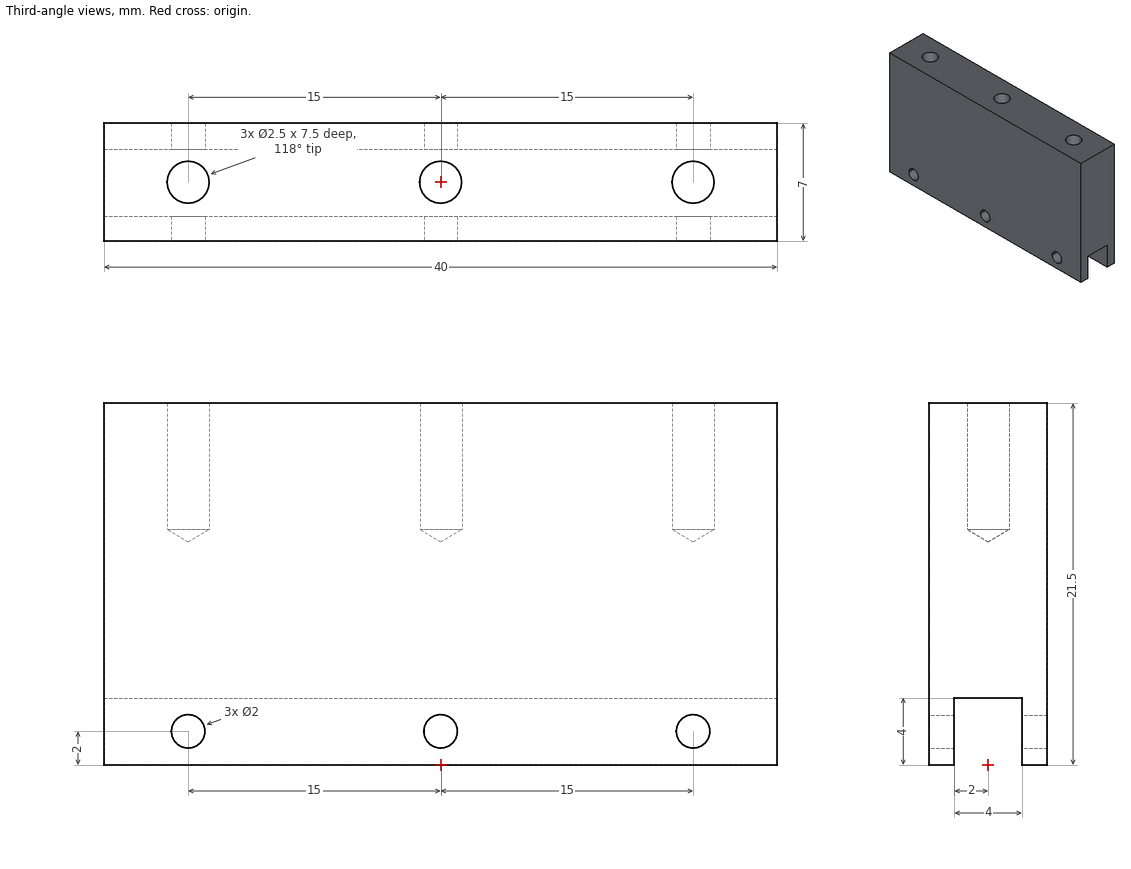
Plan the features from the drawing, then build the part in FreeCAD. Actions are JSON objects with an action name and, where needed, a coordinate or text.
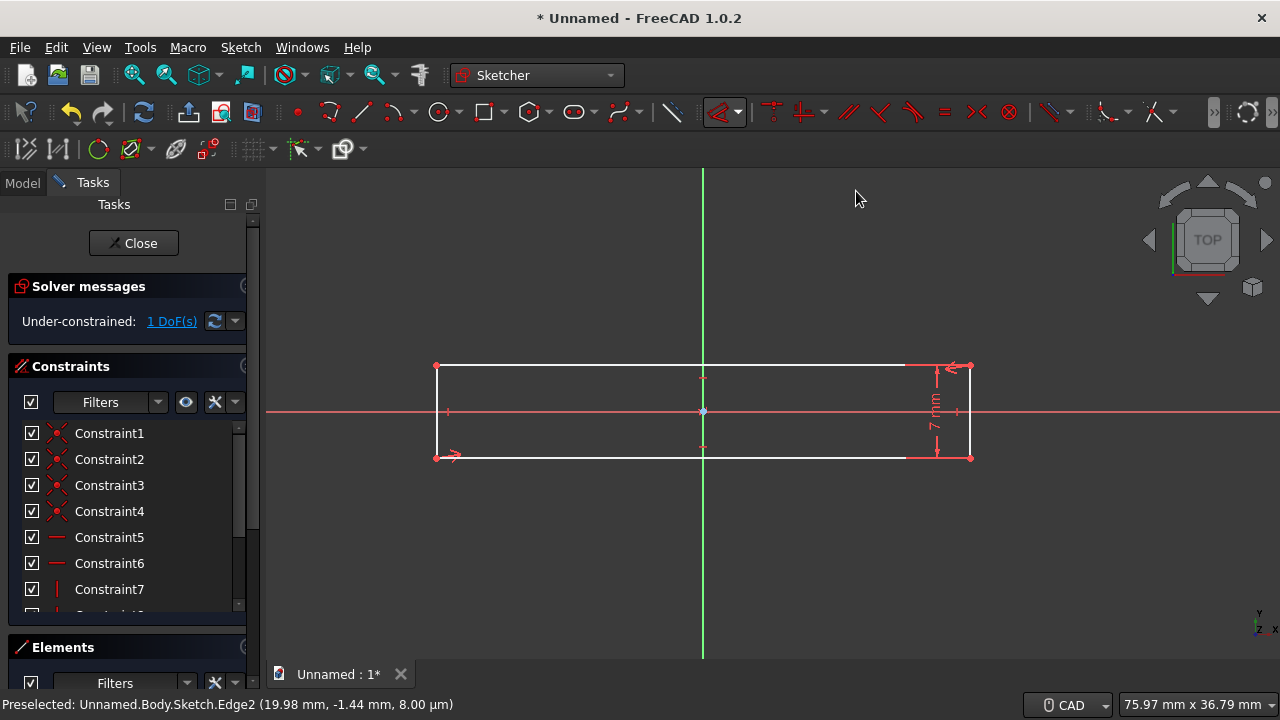
{"action": "left_click", "coordinate": [597, 458]}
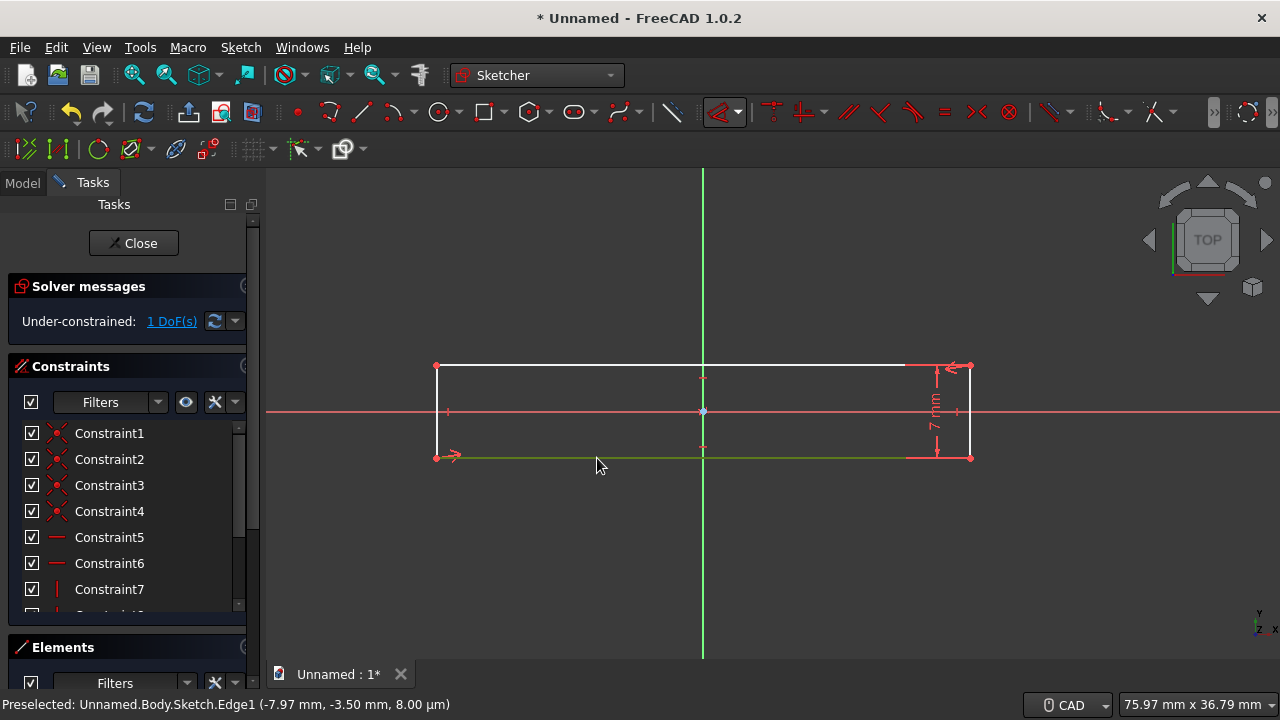
{"action": "left_click", "coordinate": [740, 112]}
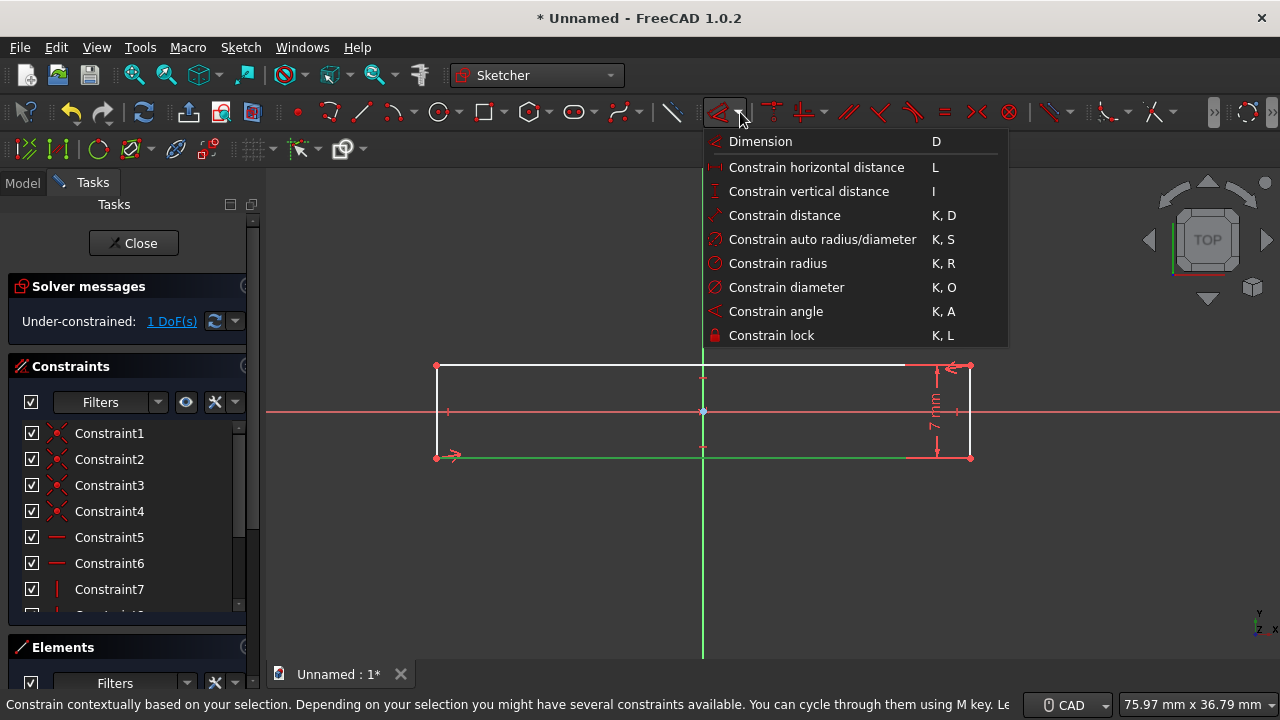
{"action": "left_click", "coordinate": [856, 167]}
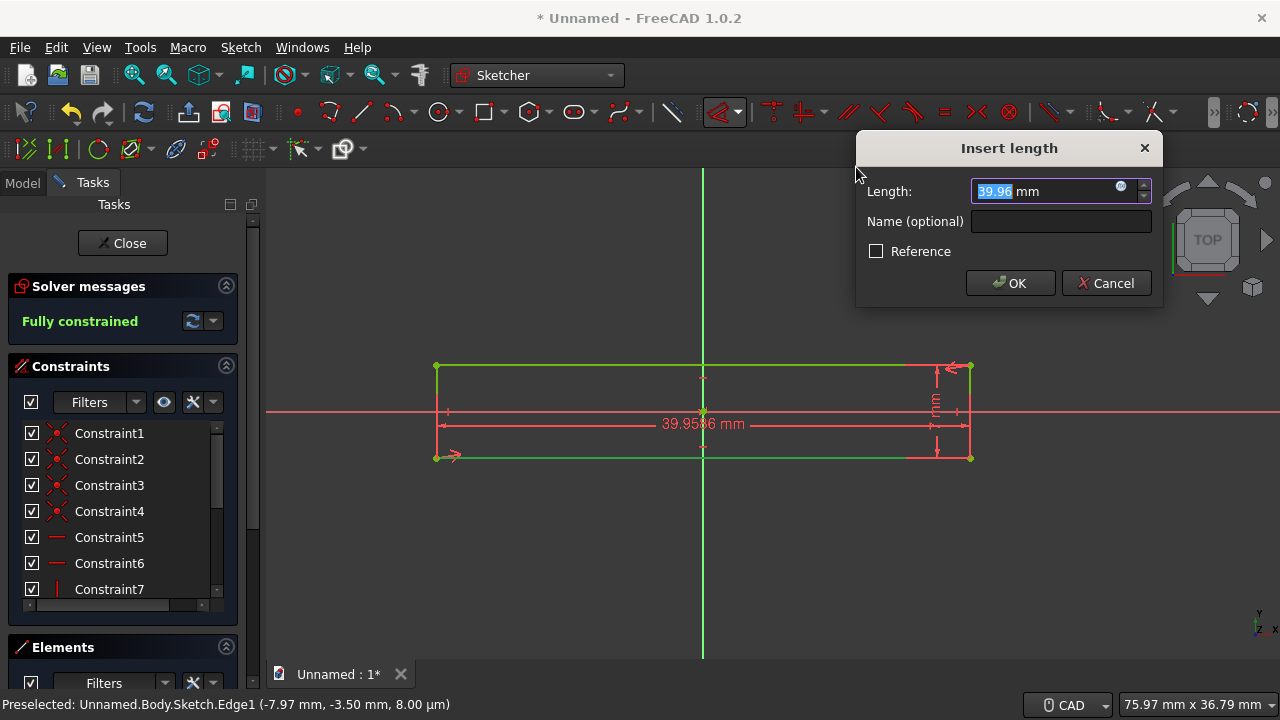
{"action": "type", "text": "40"}
{"action": "key", "text": "Return"}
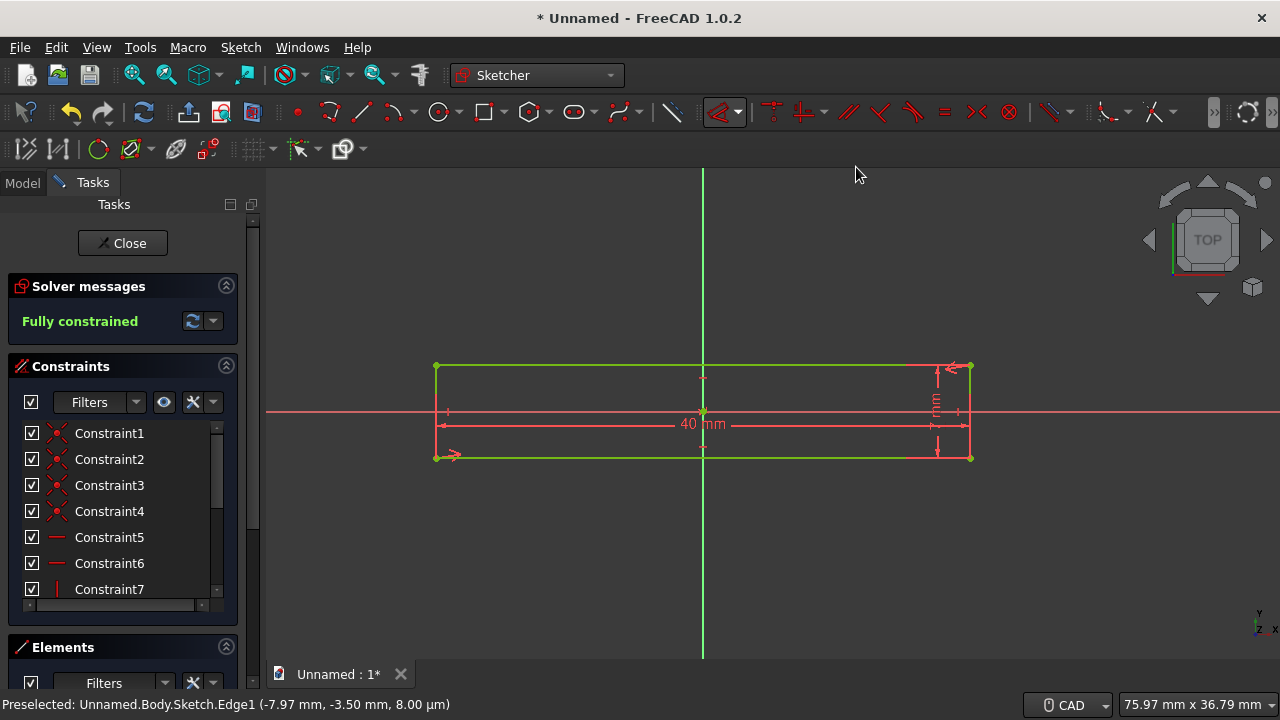
{"action": "left_click", "coordinate": [123, 243]}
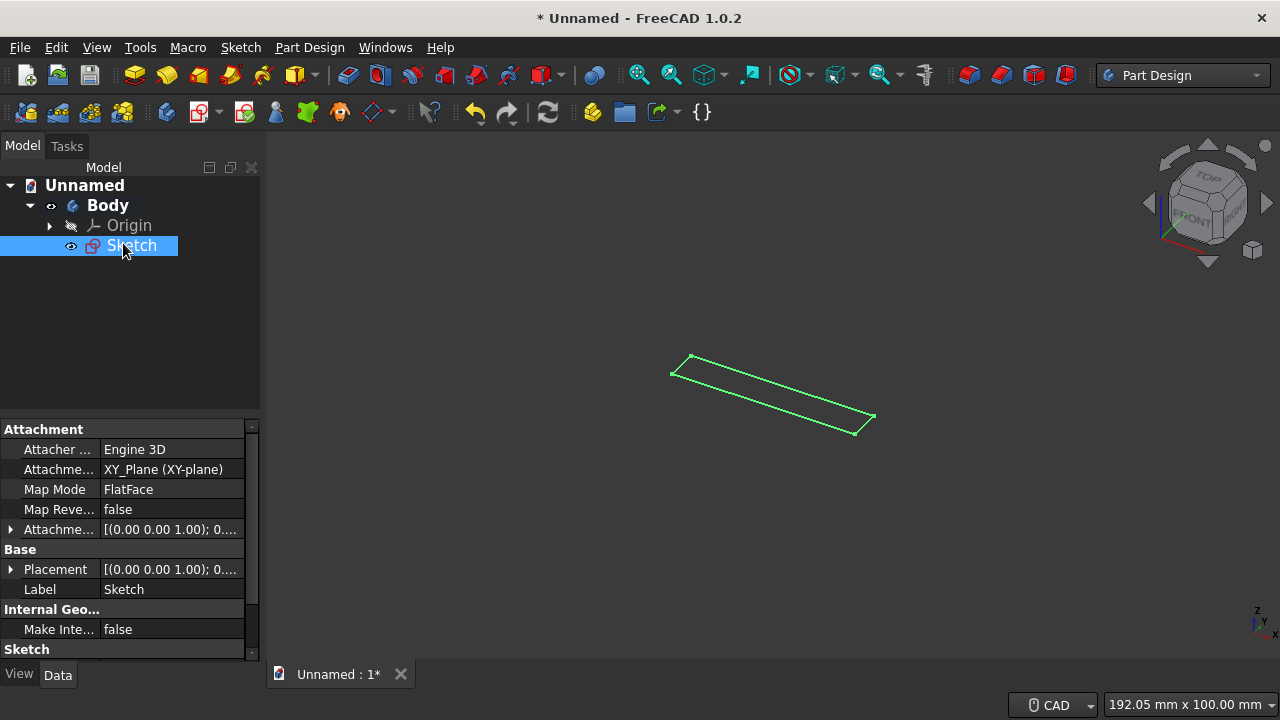
{"action": "left_click", "coordinate": [136, 76]}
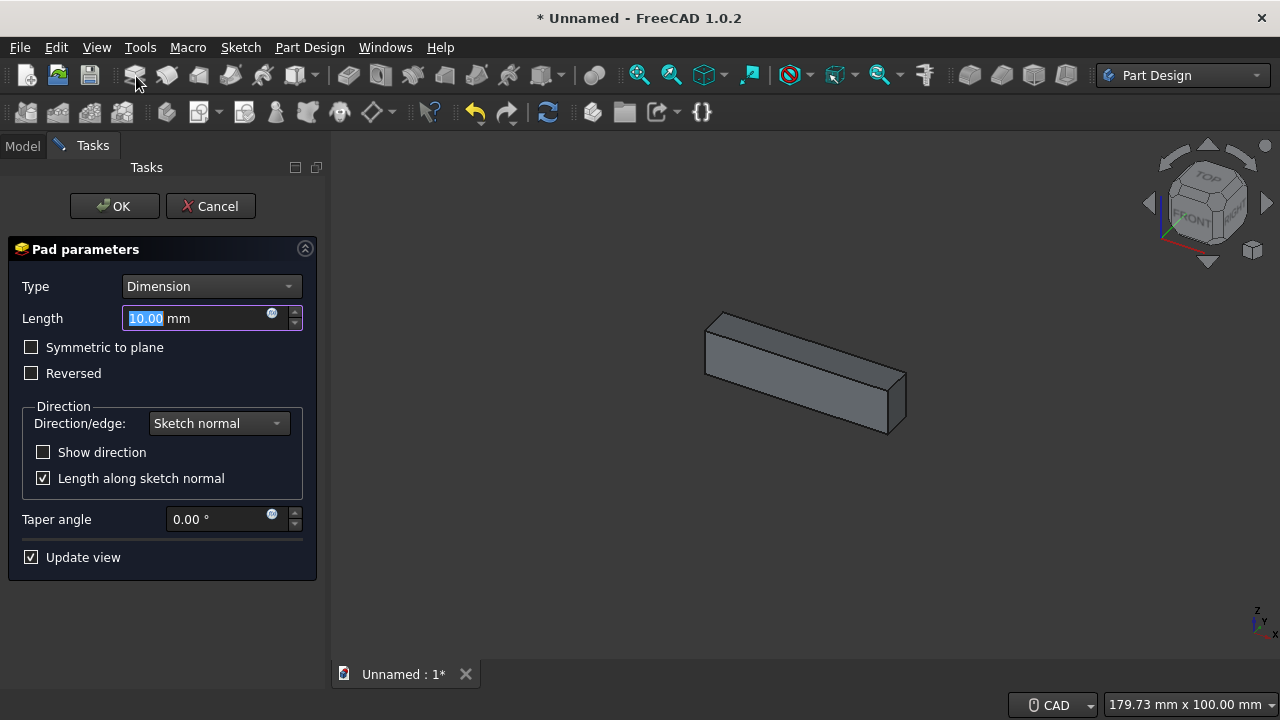
{"action": "type", "text": "21.5"}
{"action": "key", "text": "Tab"}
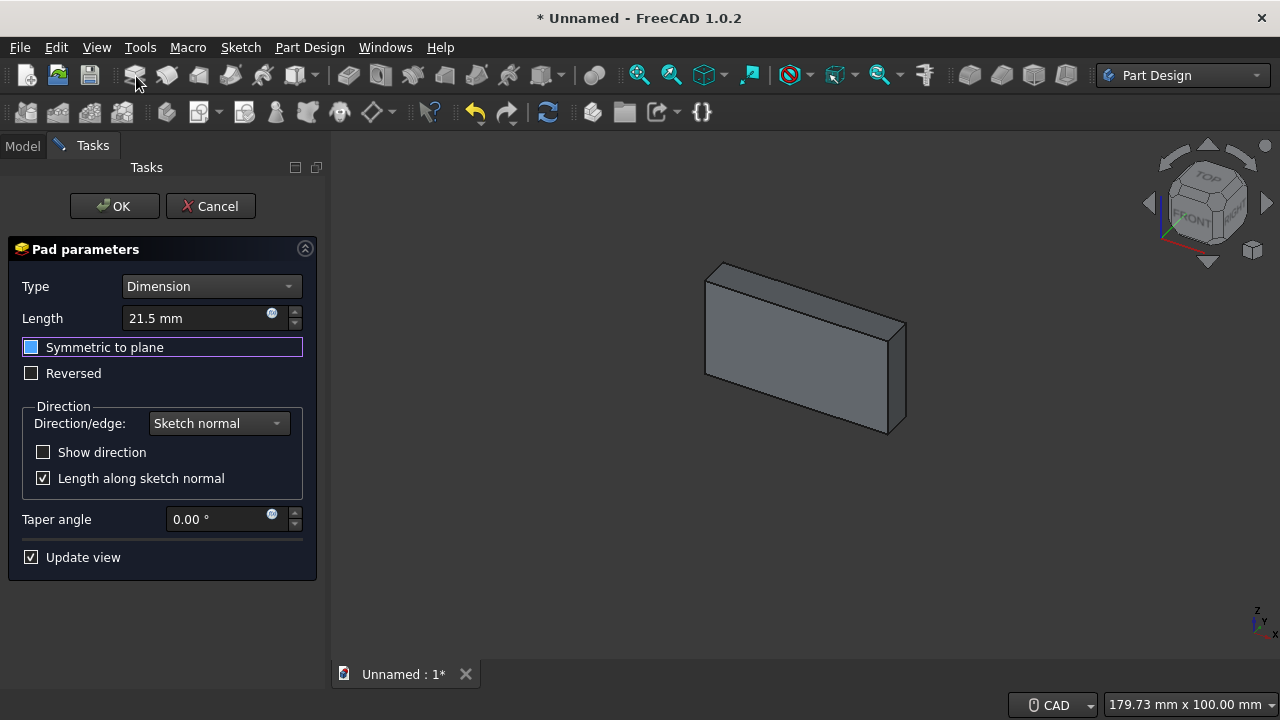
{"action": "left_click", "coordinate": [115, 206]}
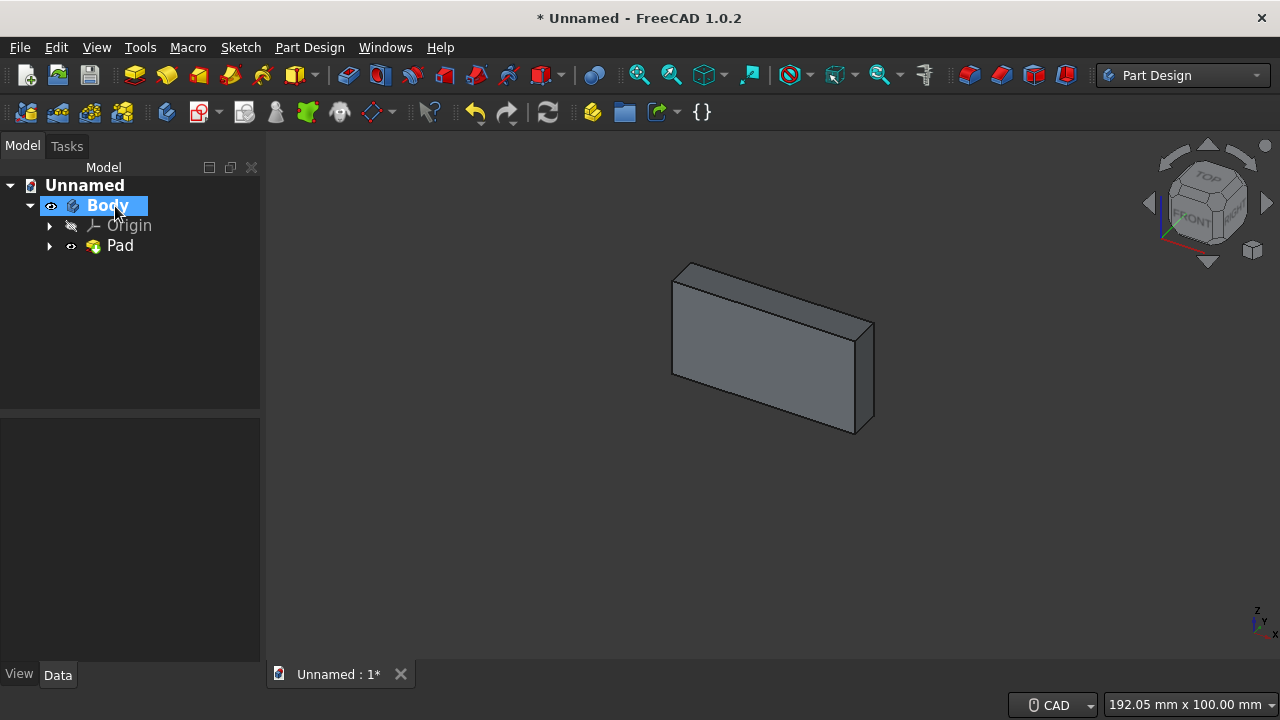
{"action": "left_click", "coordinate": [640, 76]}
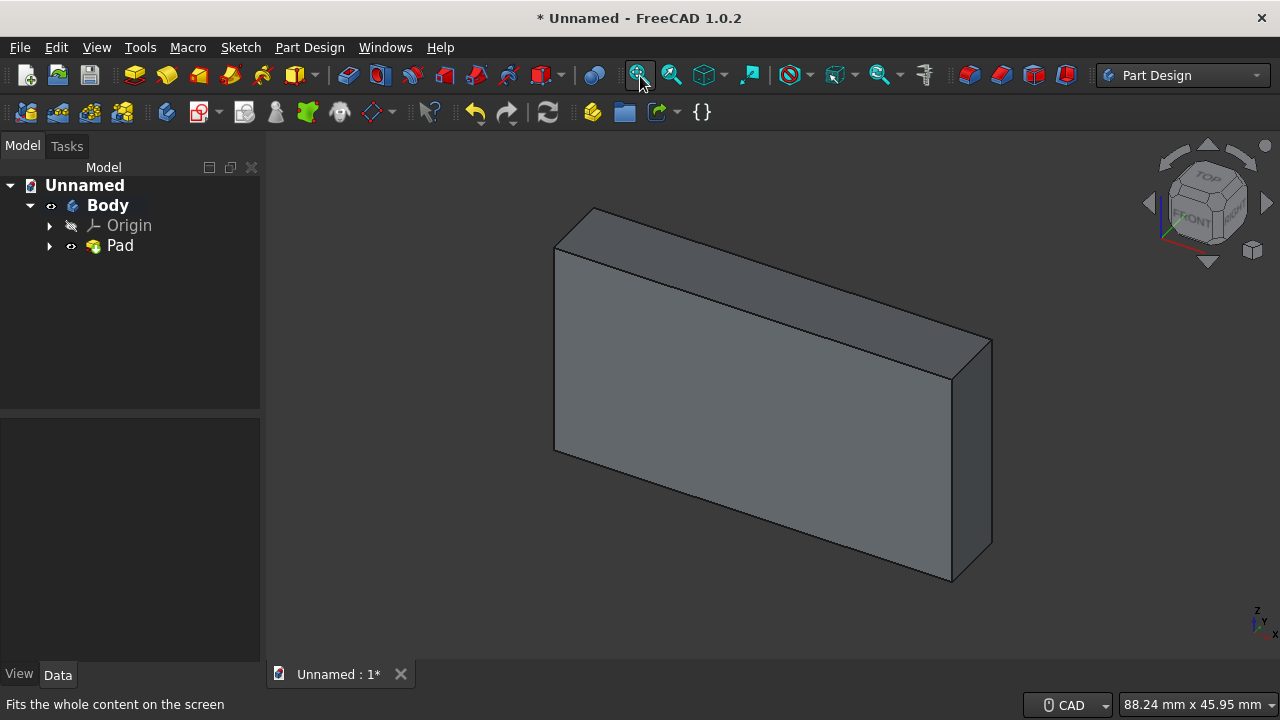
{"action": "left_click", "coordinate": [887, 330]}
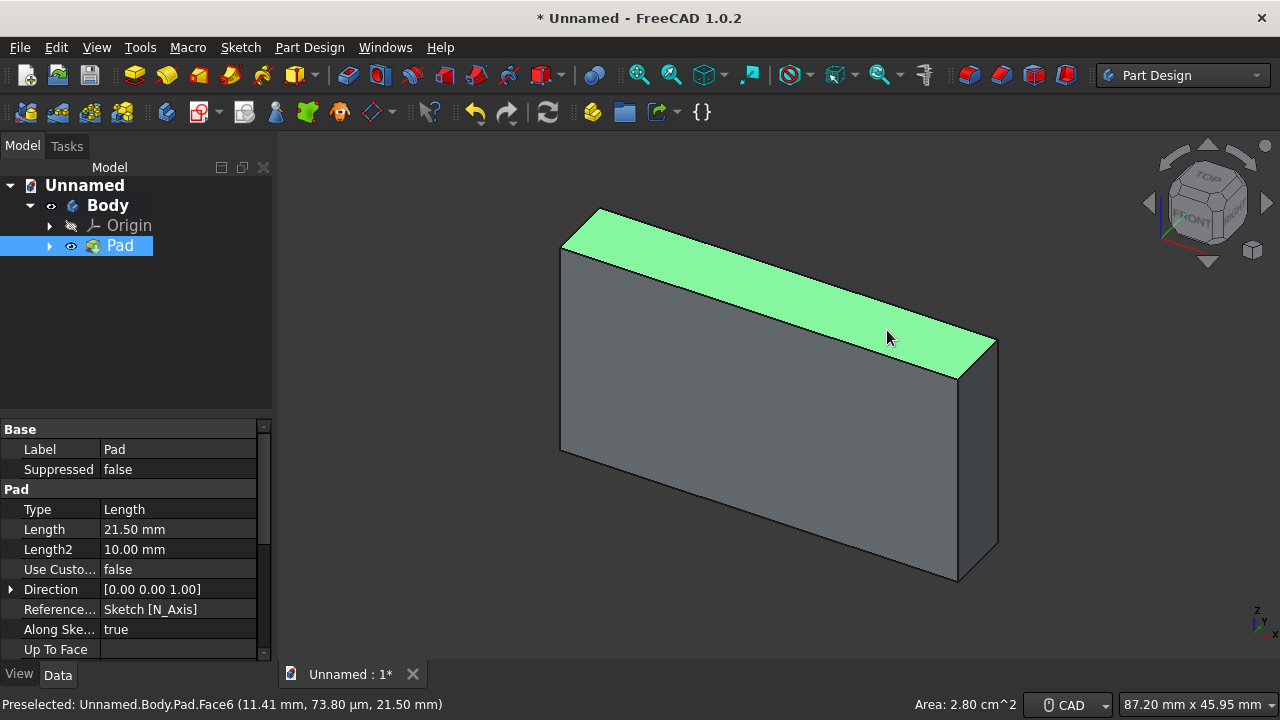
{"action": "left_click", "coordinate": [200, 112]}